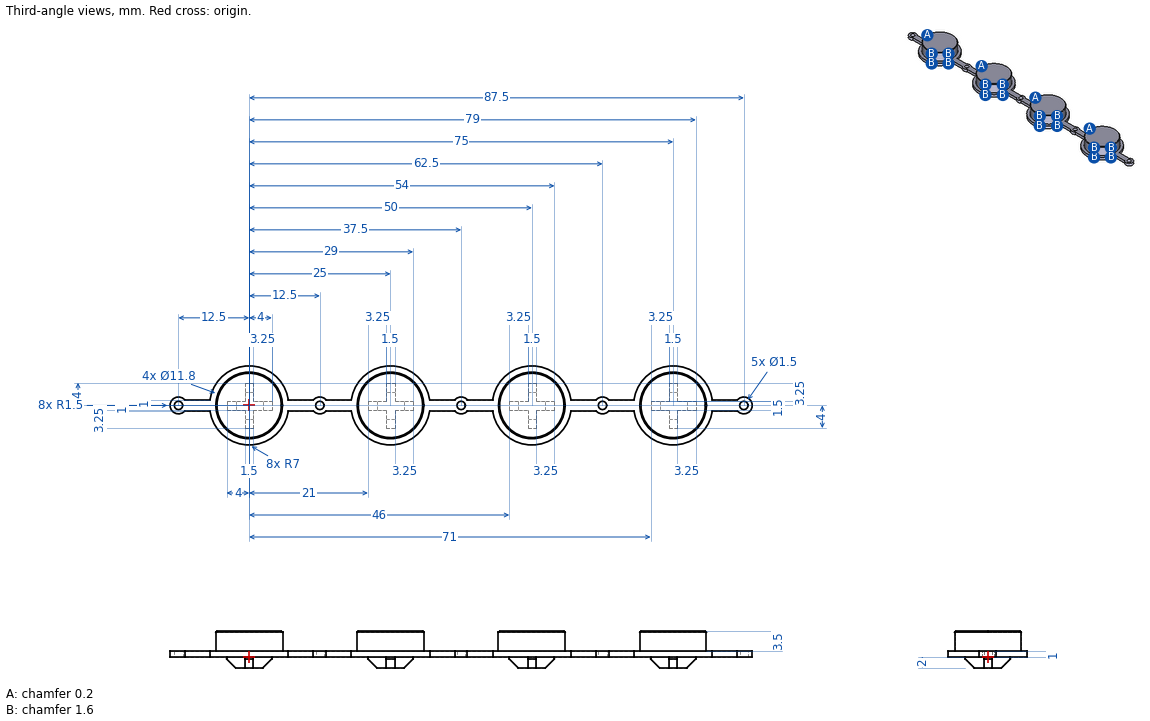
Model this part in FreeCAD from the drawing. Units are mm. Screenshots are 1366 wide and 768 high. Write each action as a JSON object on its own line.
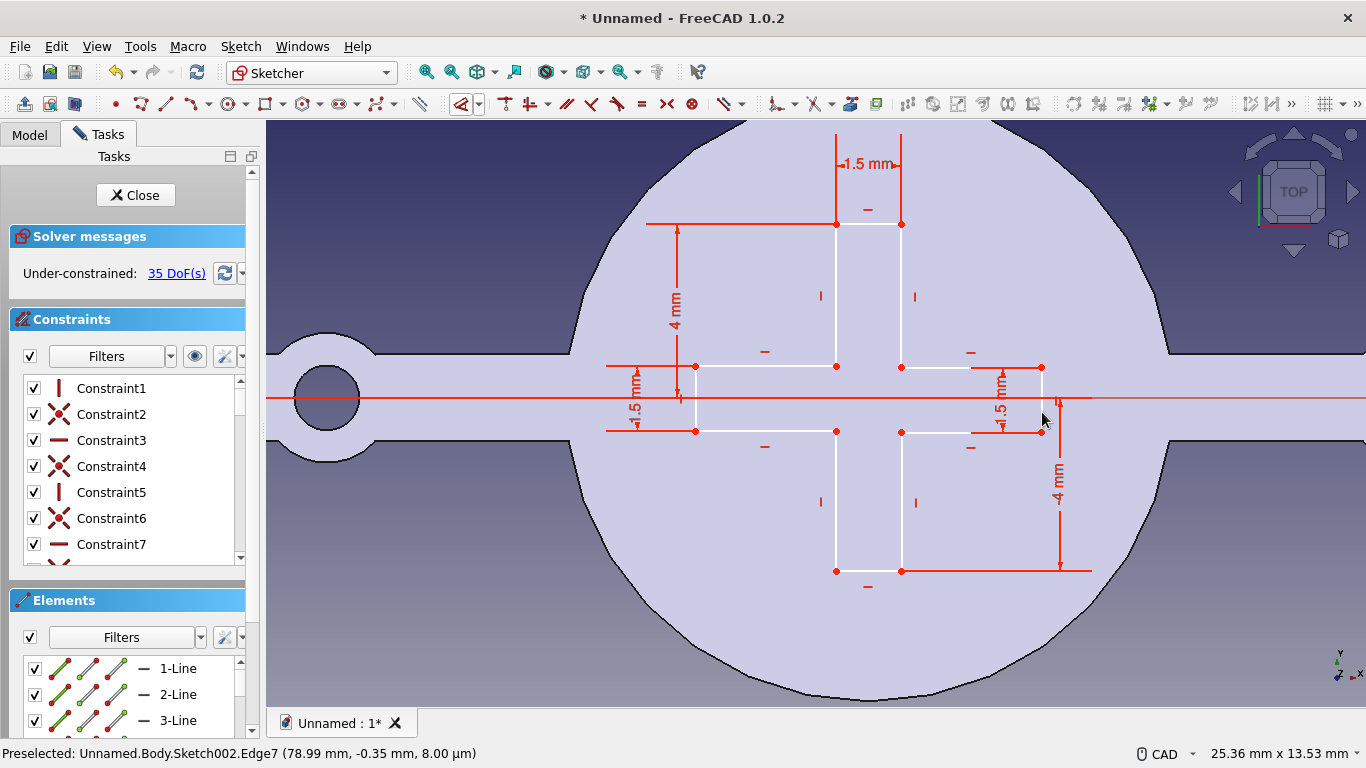
{"action": "left_click", "coordinate": [882, 571]}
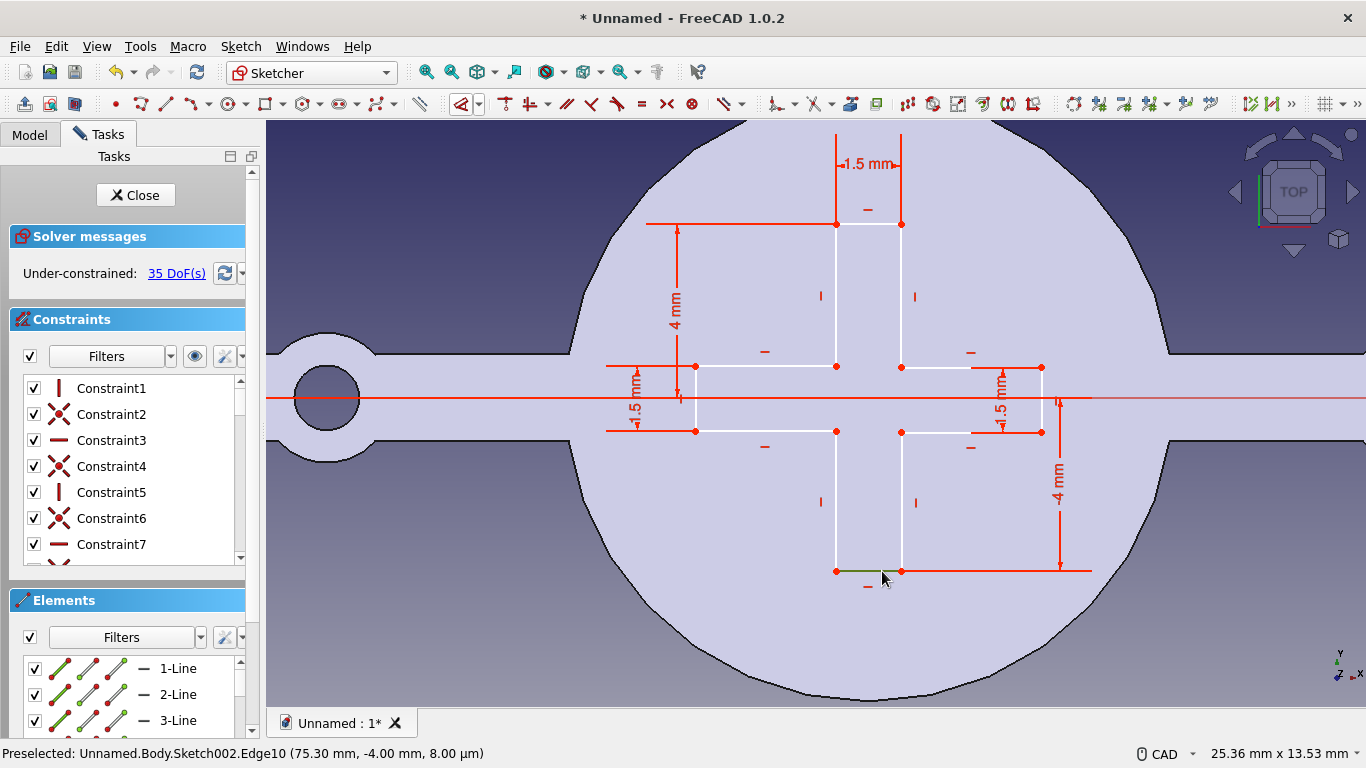
{"action": "key", "text": "l"}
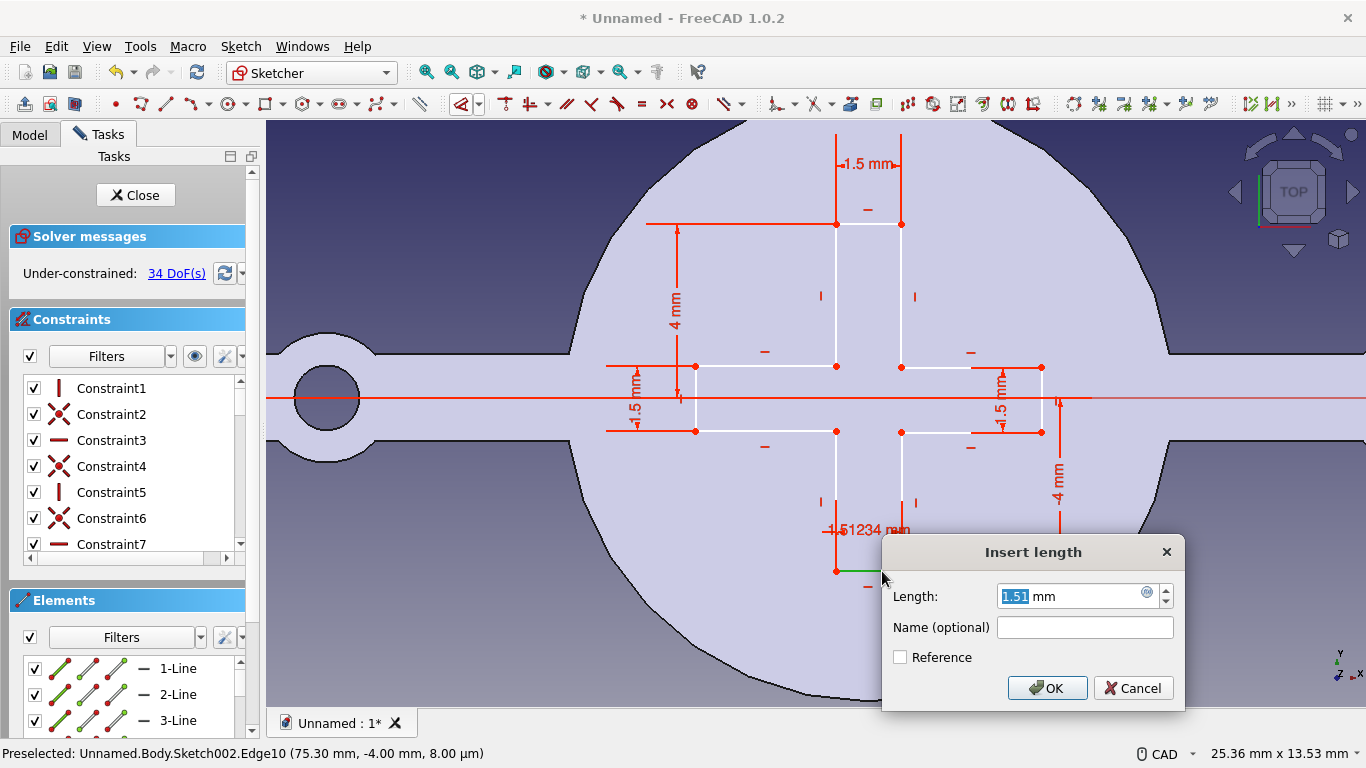
{"action": "type", "text": "1.5"}
{"action": "key", "text": "Return"}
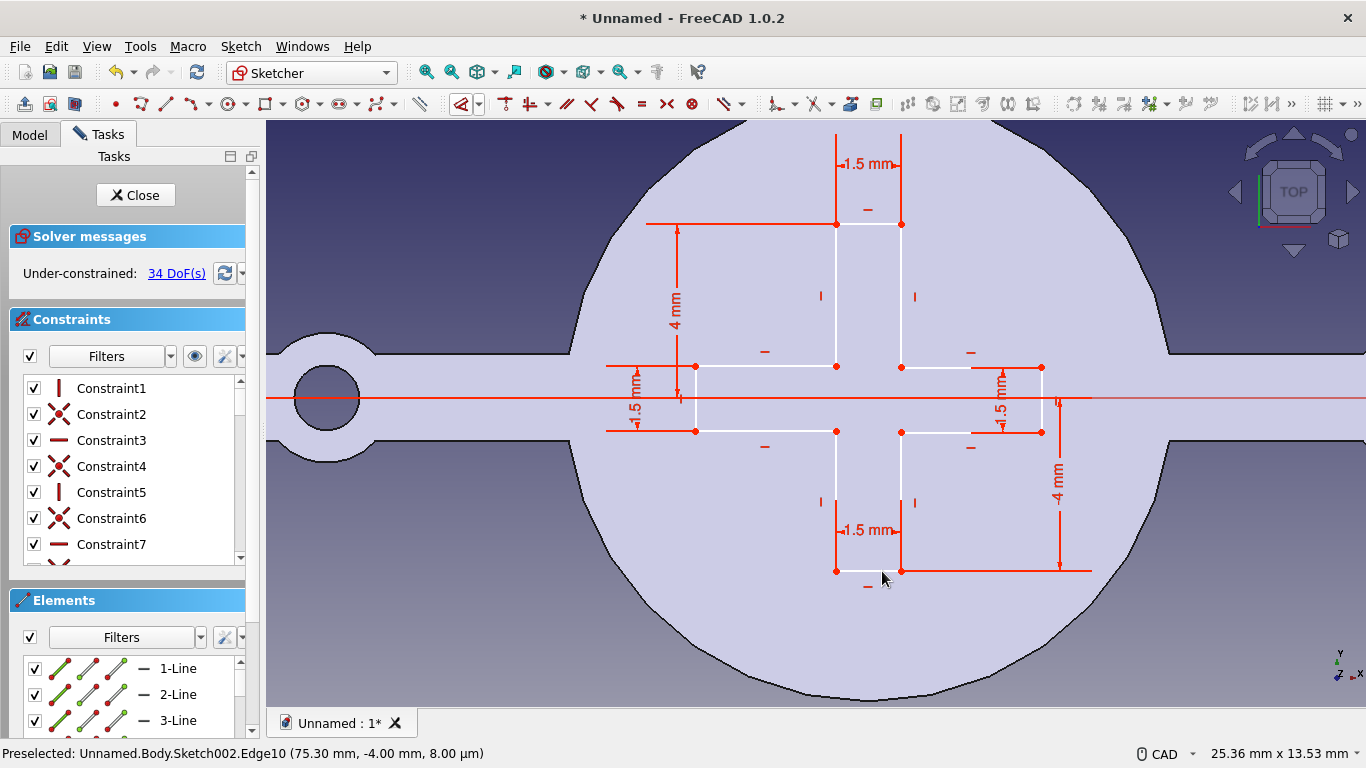
{"action": "scroll", "coordinate": [1046, 417], "scroll_direction": "down", "scroll_amount": 9}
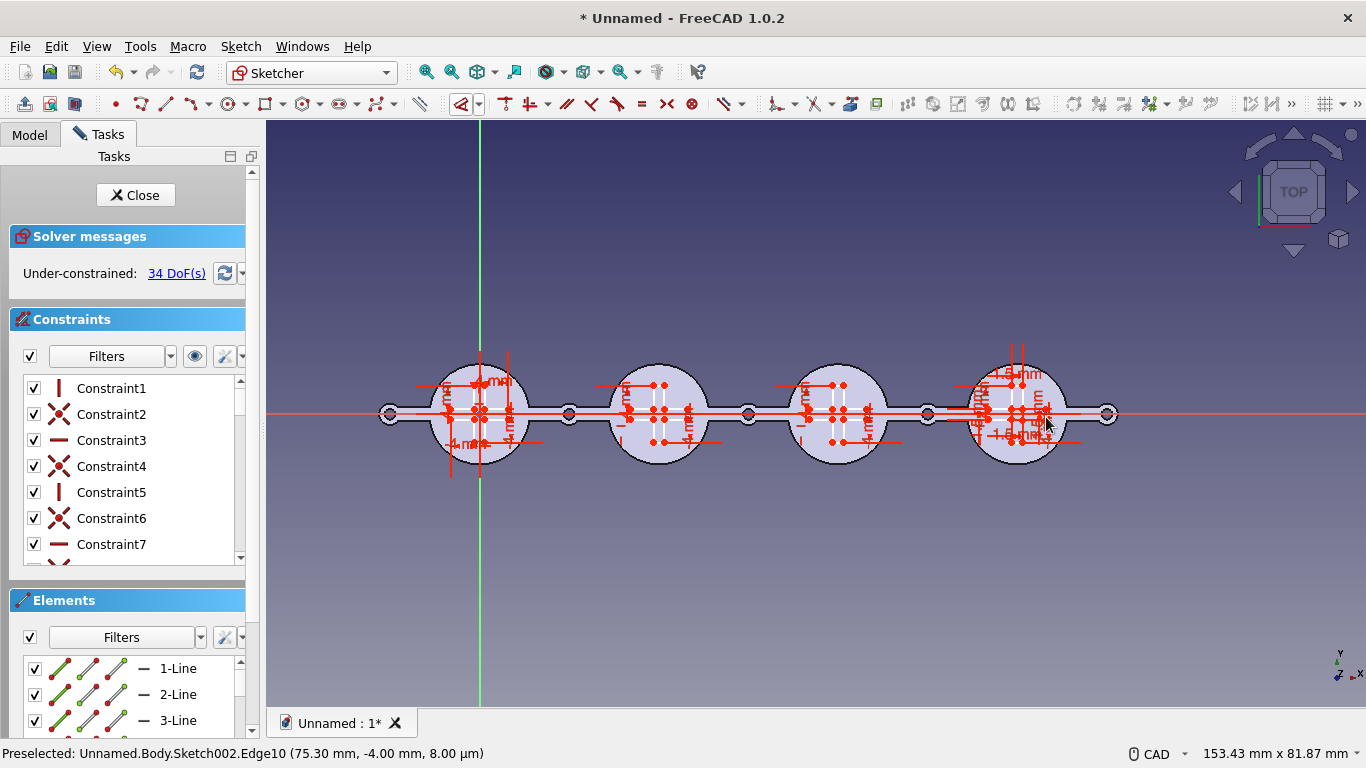
{"action": "scroll", "coordinate": [809, 417], "scroll_direction": "up", "scroll_amount": 9}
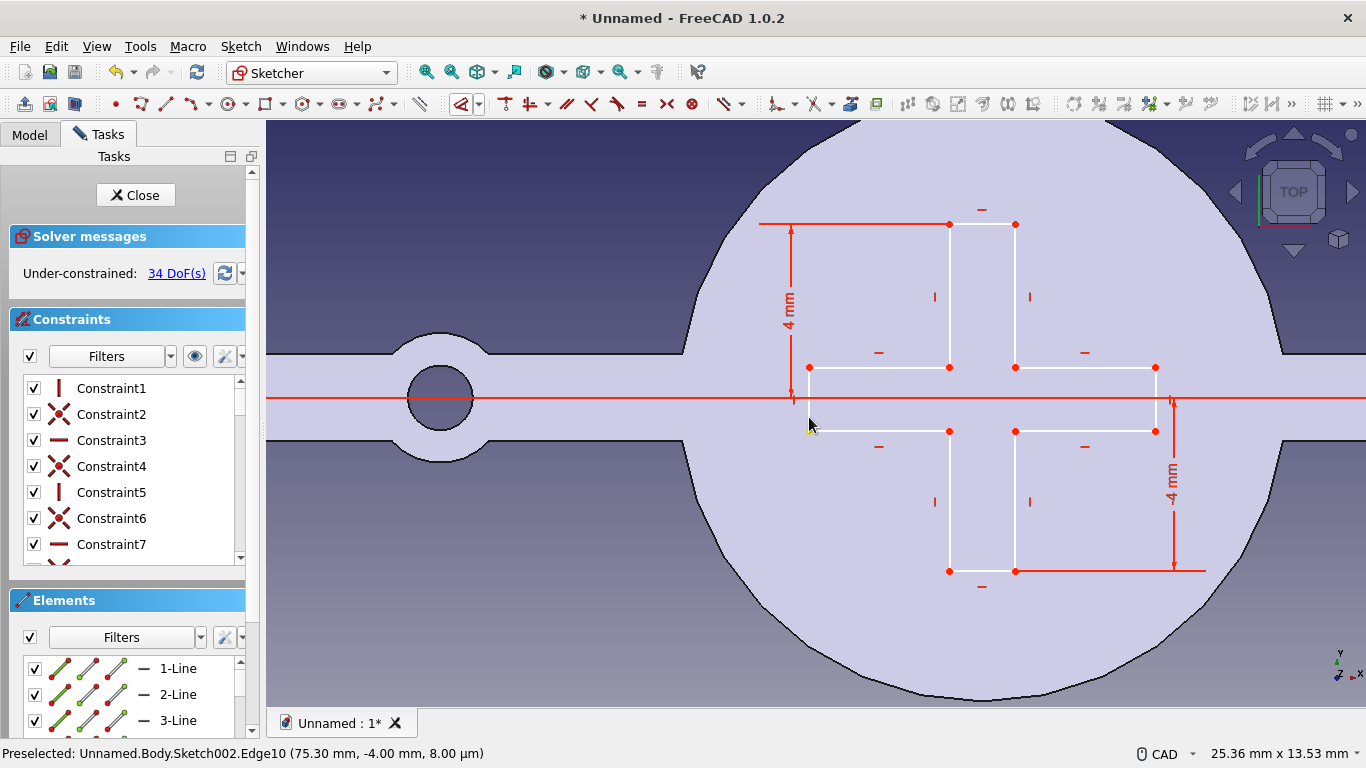
{"action": "left_click", "coordinate": [809, 412]}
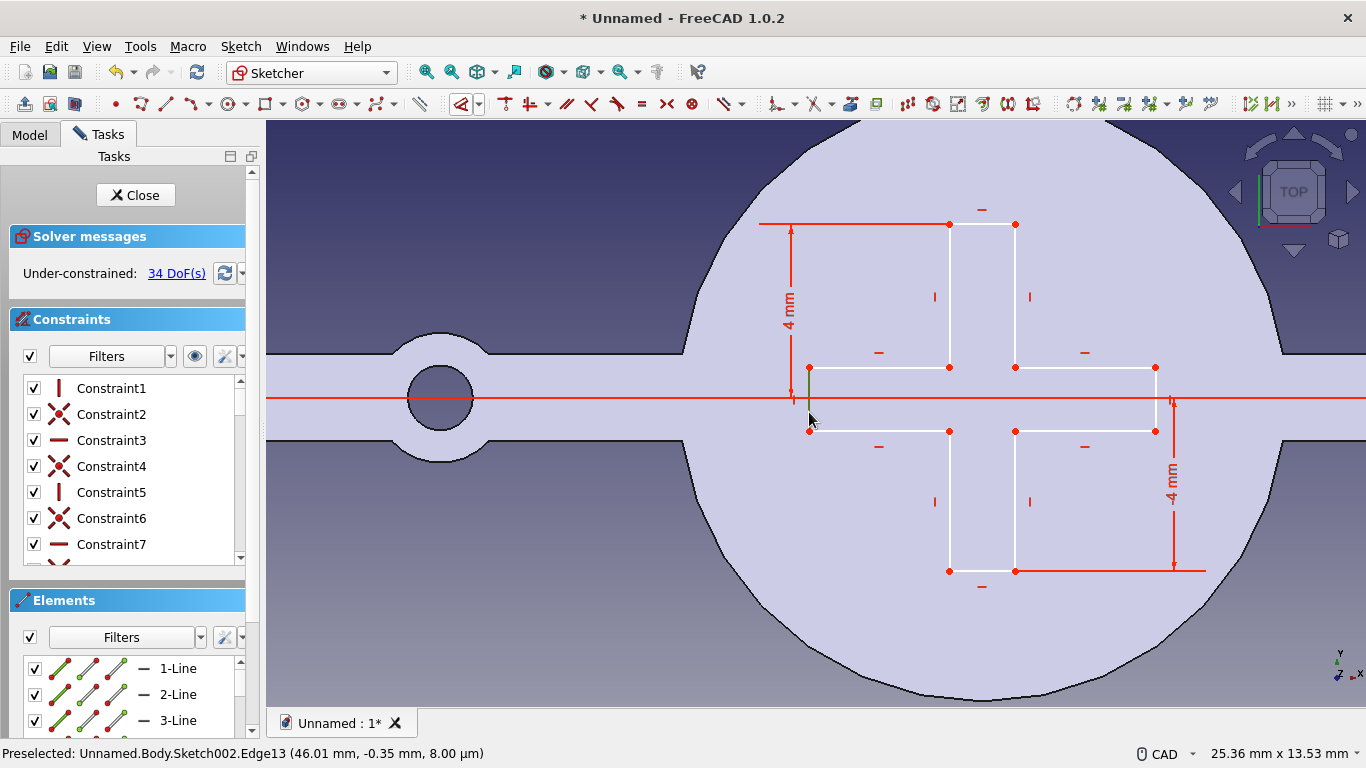
{"action": "key", "text": "i"}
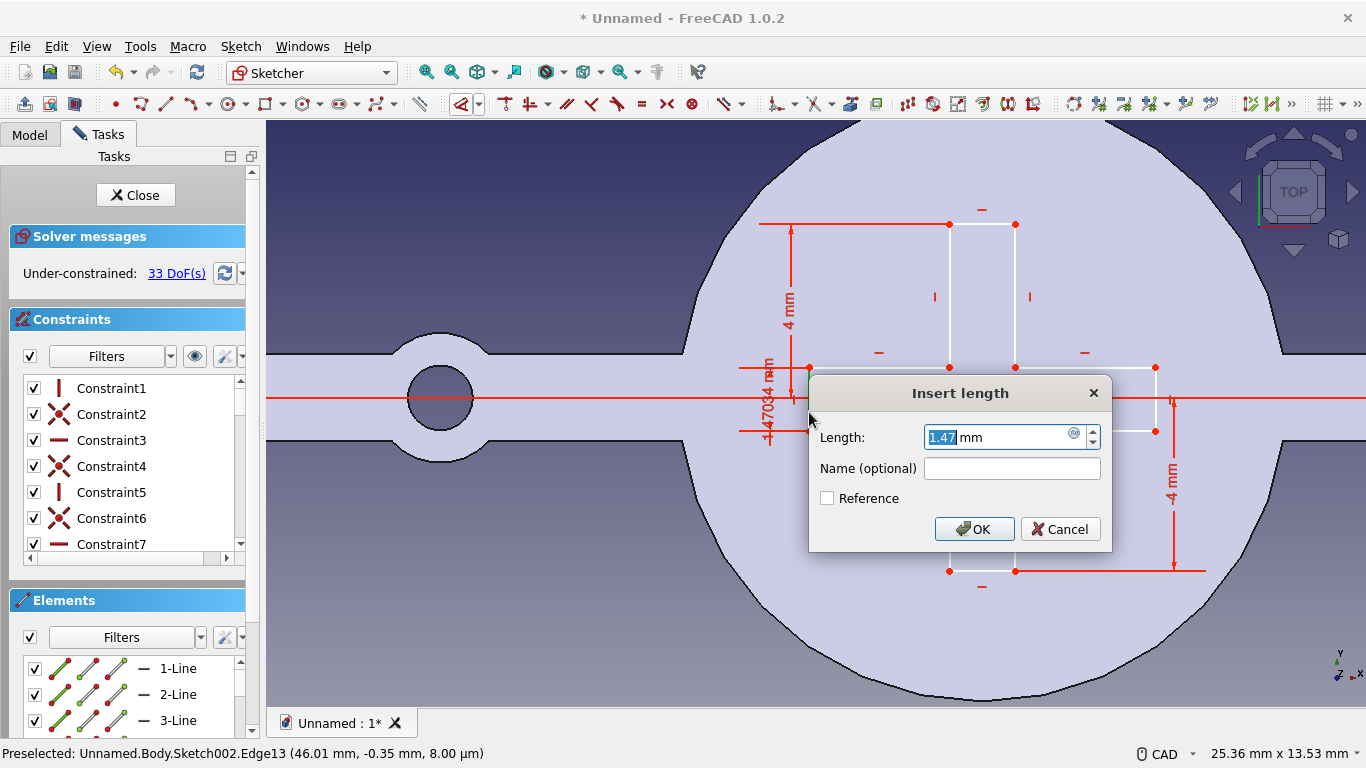
{"action": "type", "text": "1.5"}
{"action": "key", "text": "Return"}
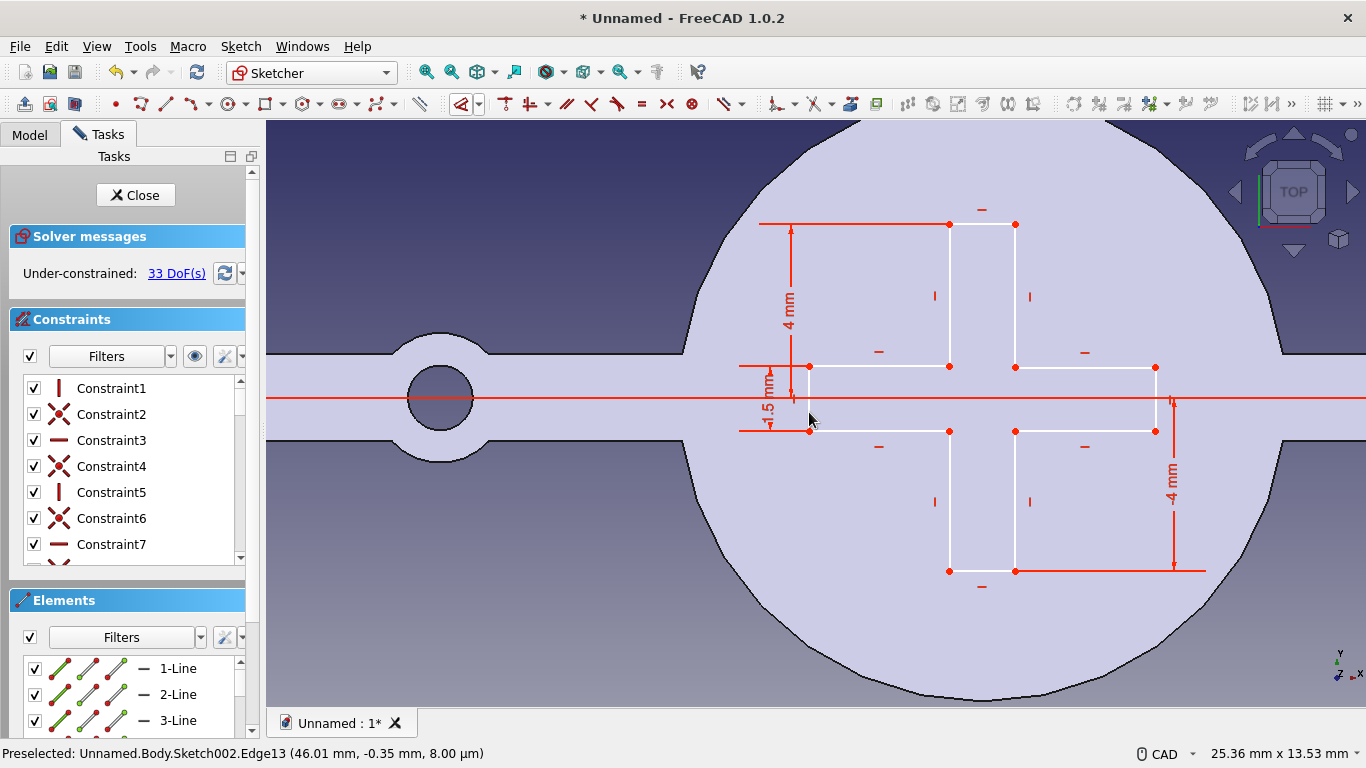
{"action": "left_click", "coordinate": [969, 224]}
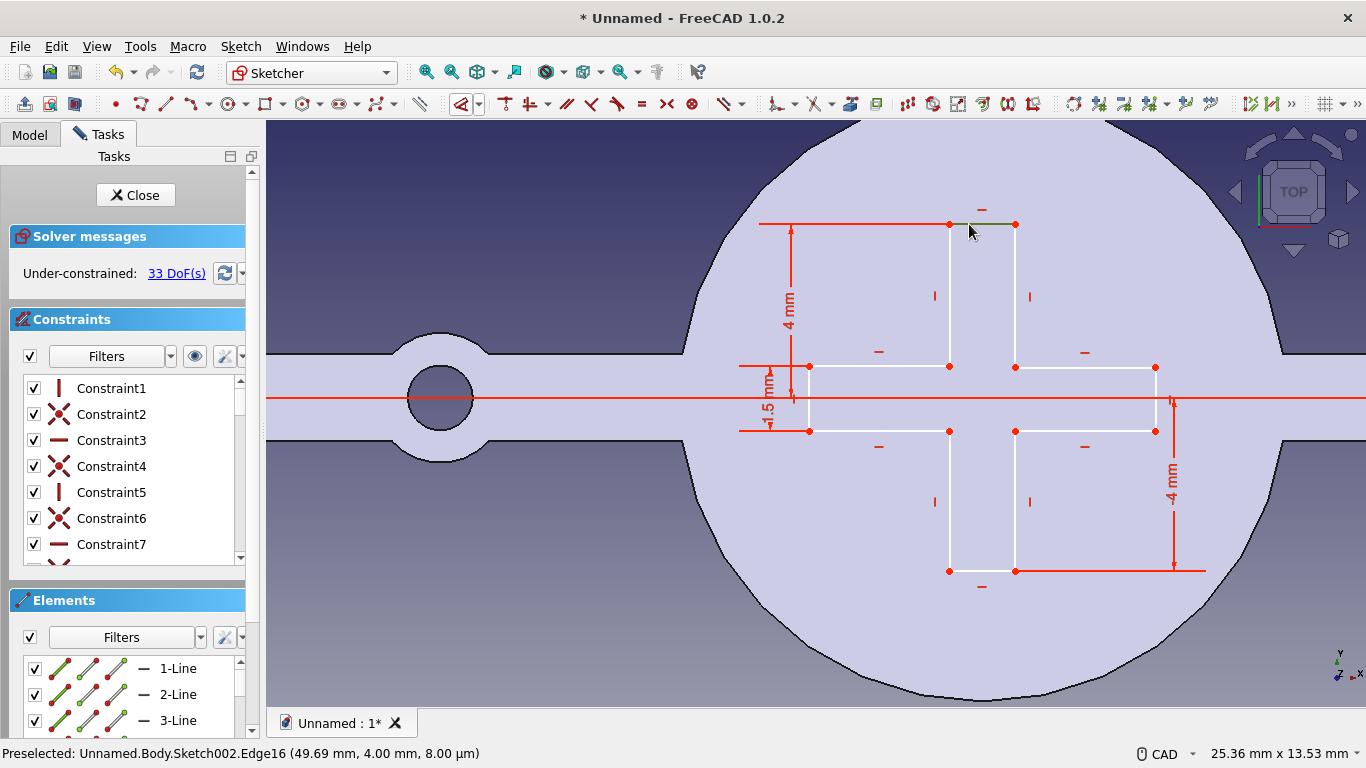
{"action": "key", "text": "l"}